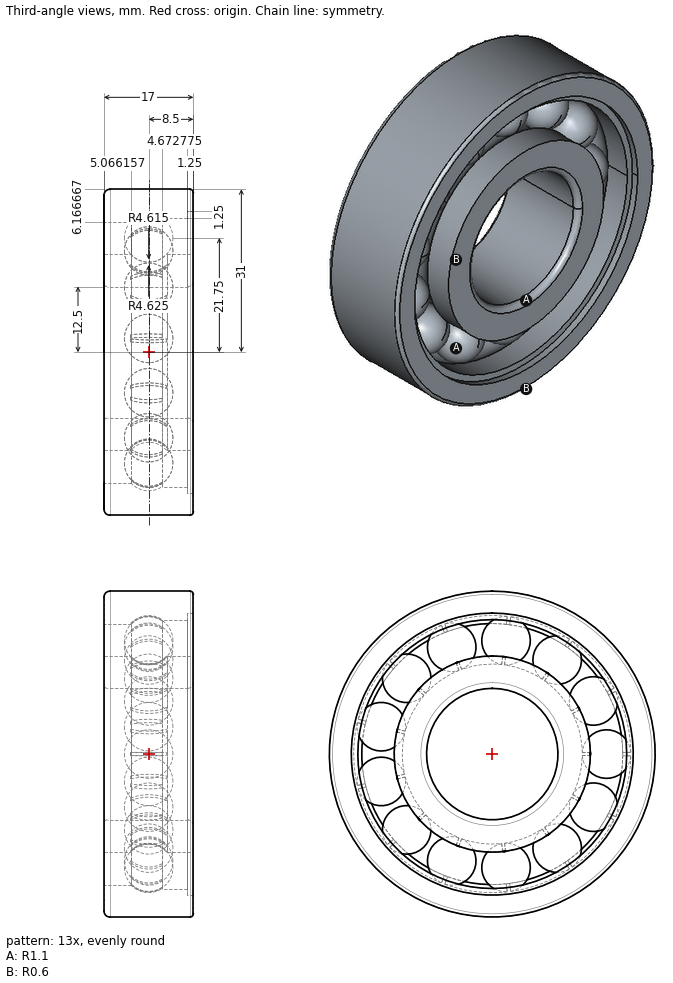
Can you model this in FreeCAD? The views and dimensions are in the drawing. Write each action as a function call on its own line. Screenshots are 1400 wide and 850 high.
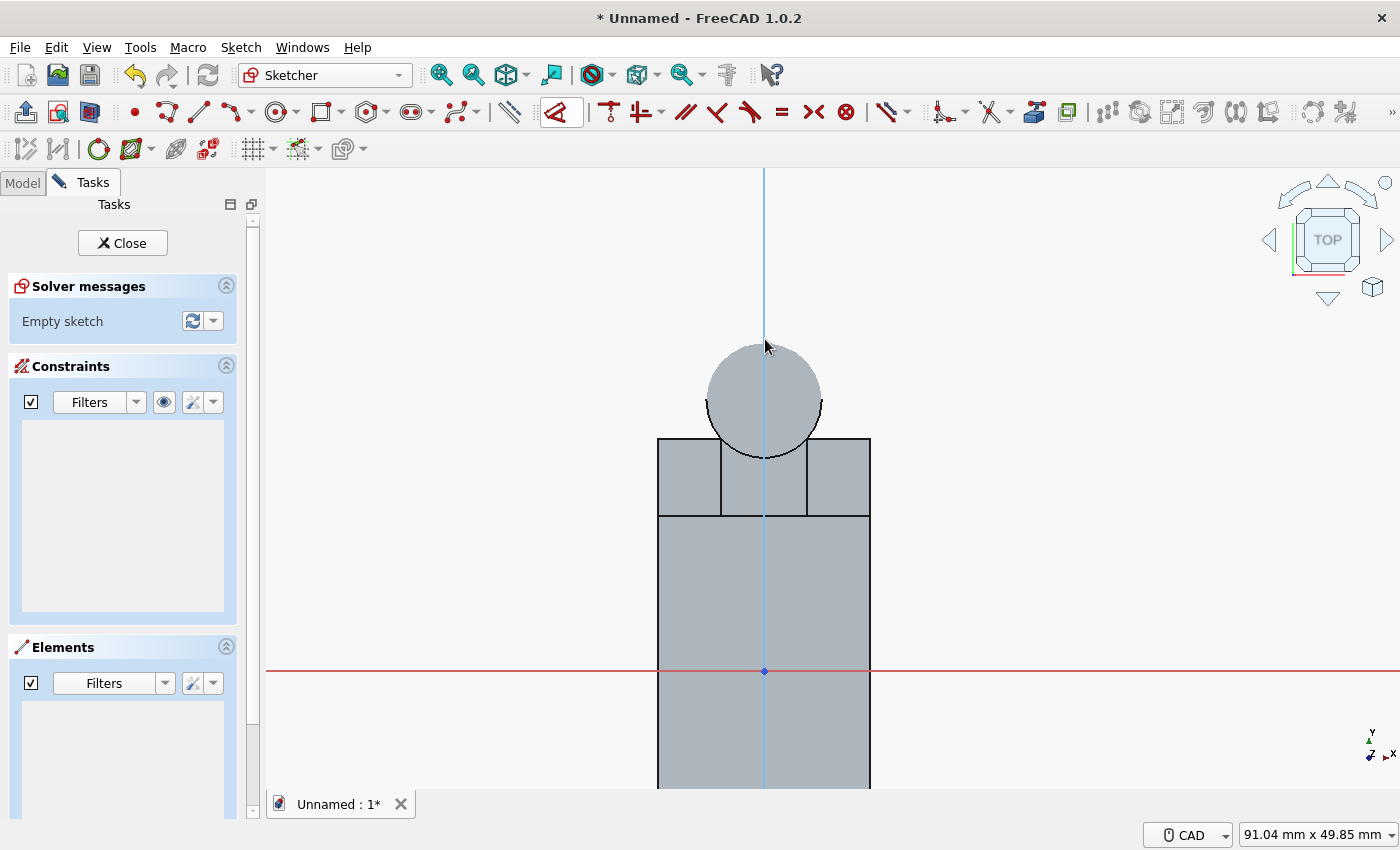
click(168, 112)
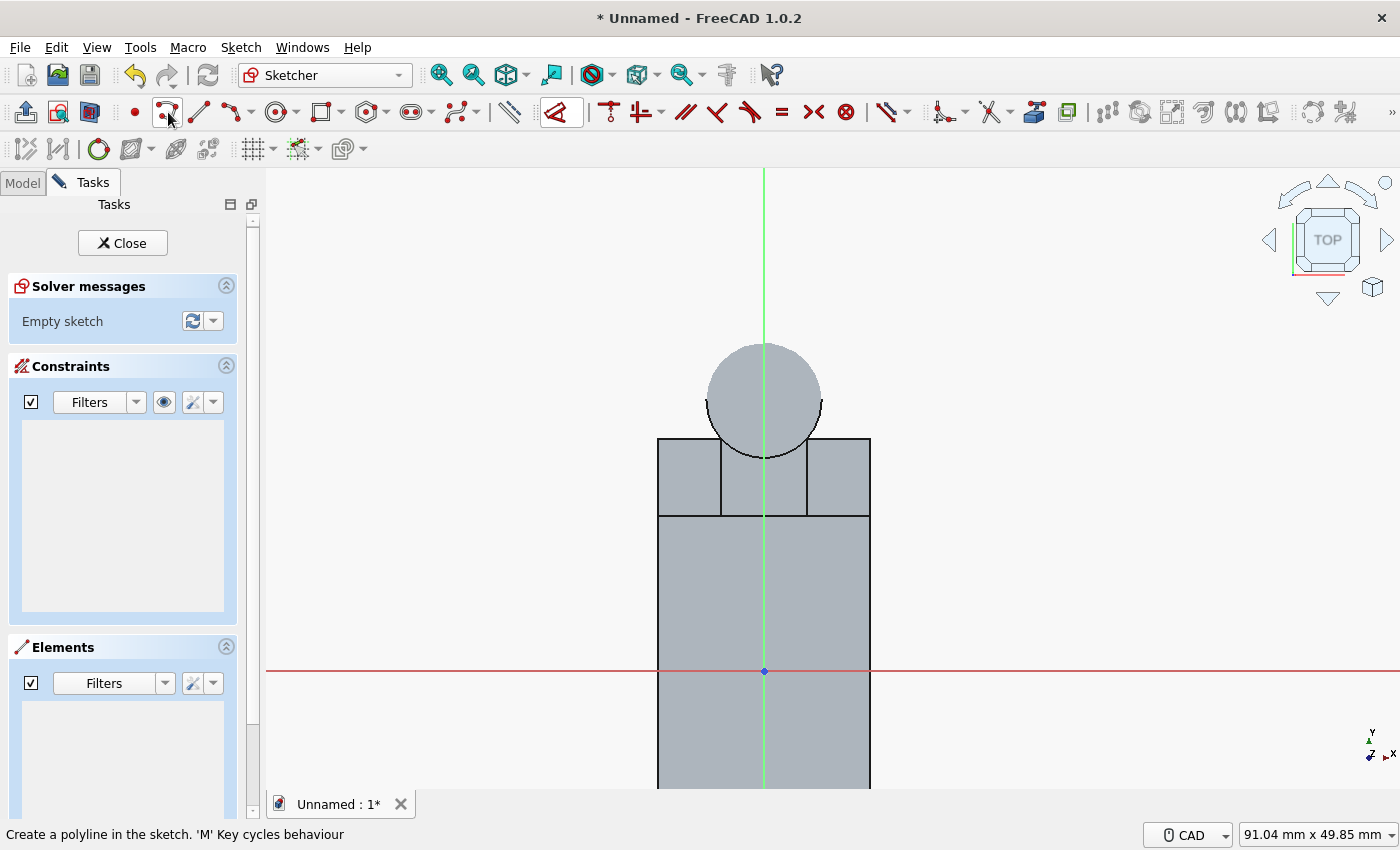
click(796, 353)
click(854, 353)
click(854, 337)
click(870, 337)
click(870, 285)
click(658, 285)
click(658, 362)
click(721, 362)
right_click(721, 362)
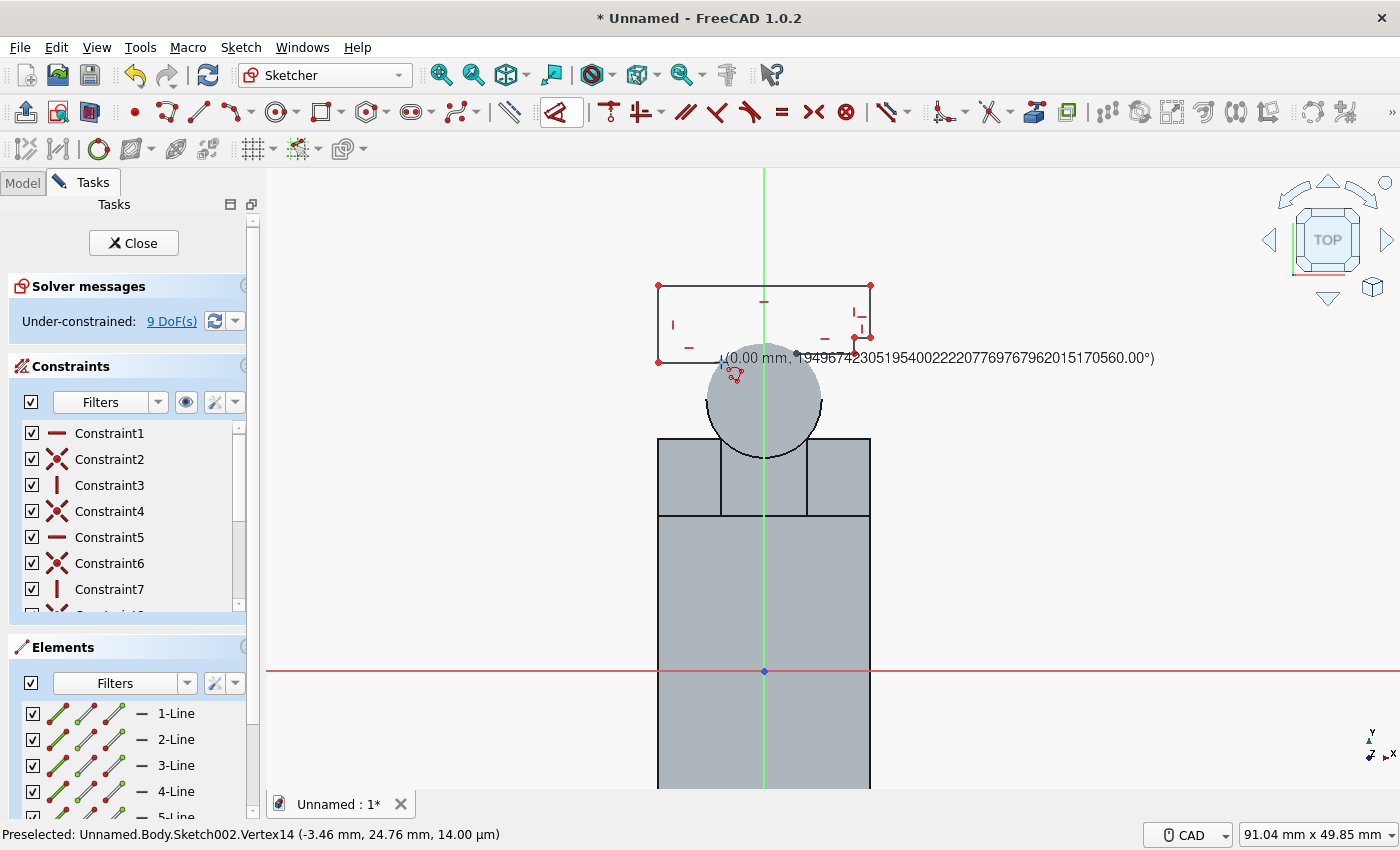
key(g)
key(3)
key(a)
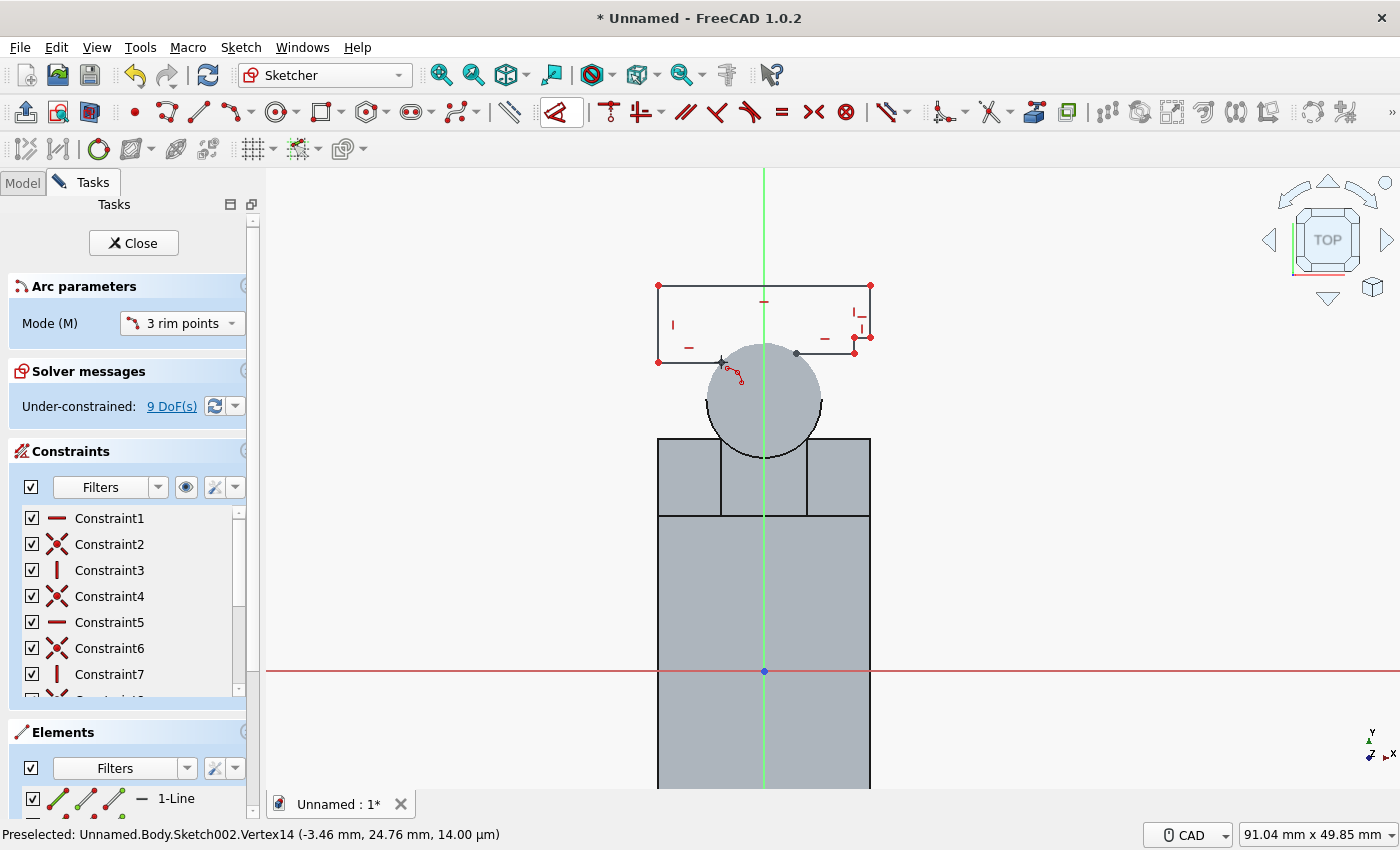
click(721, 363)
click(796, 354)
click(749, 345)
key(Escape)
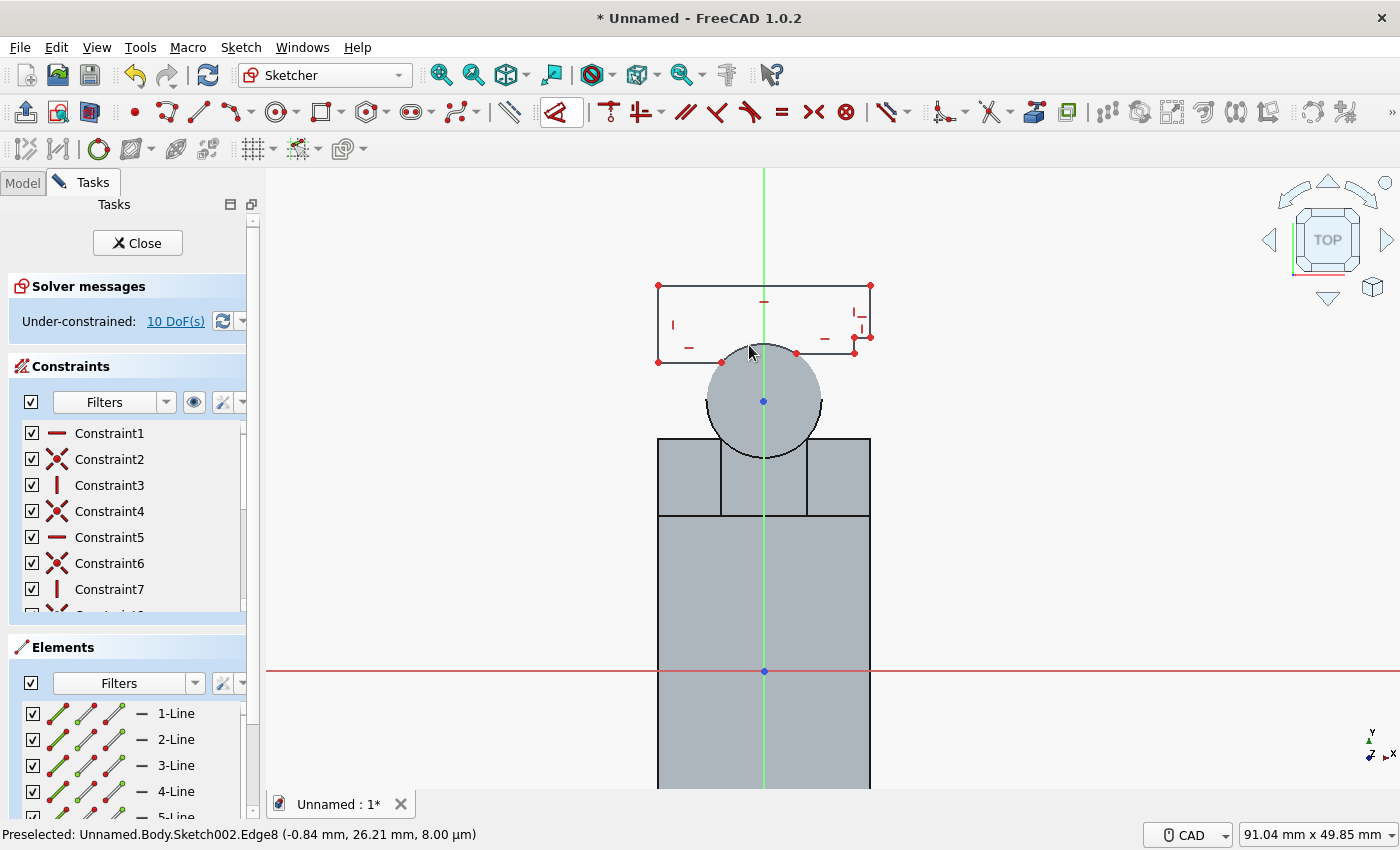
click(764, 402)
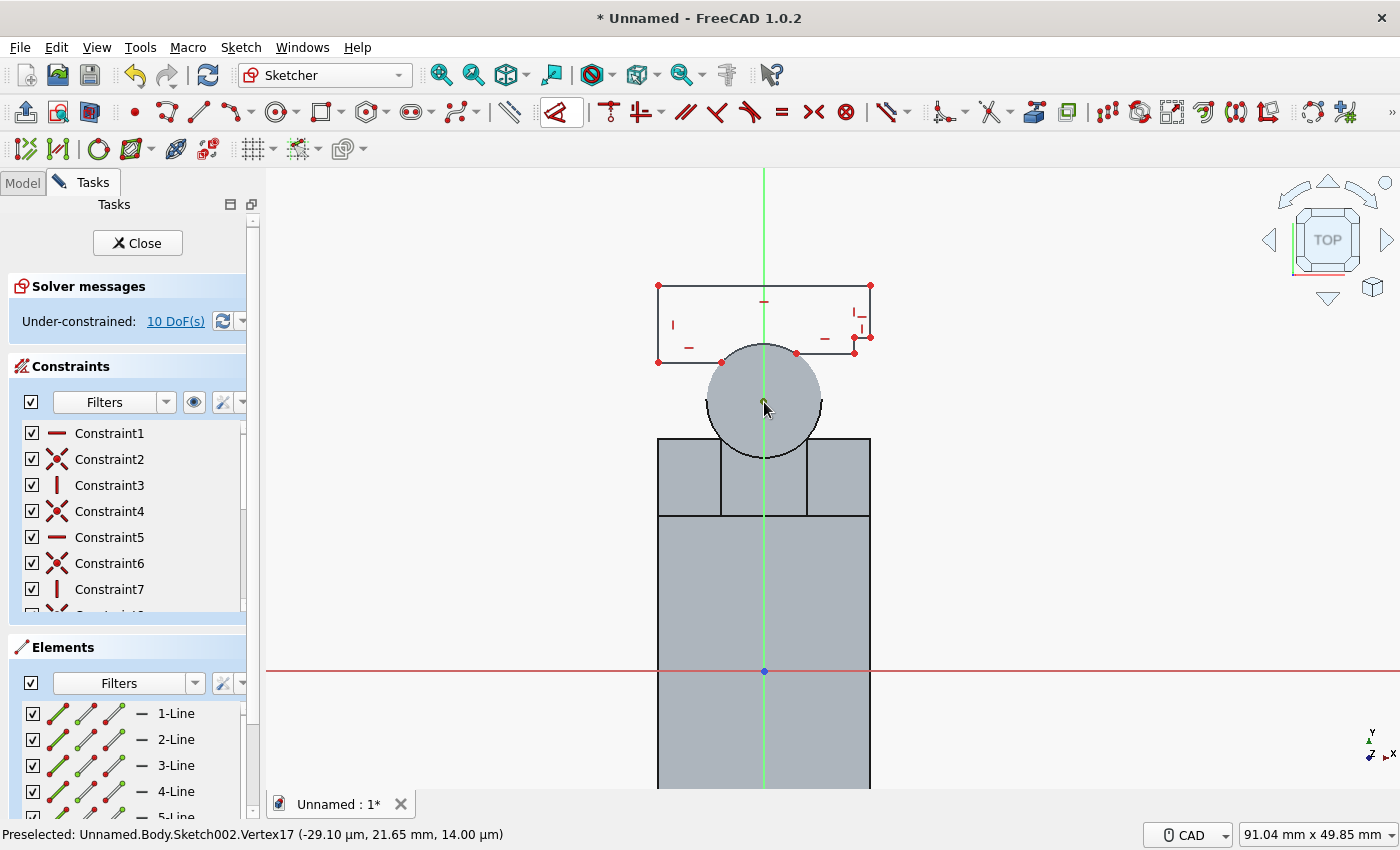
click(764, 721)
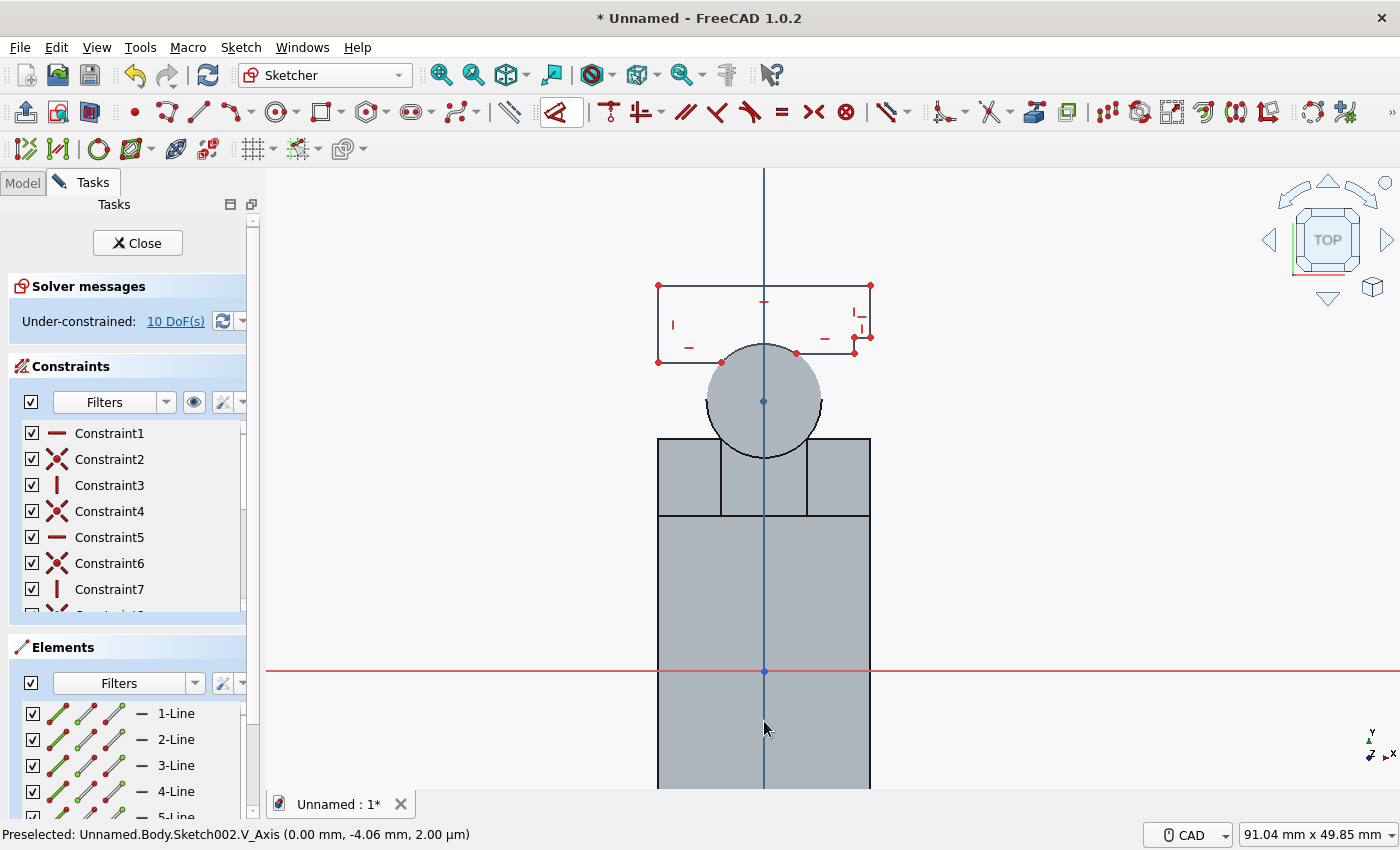
key(c)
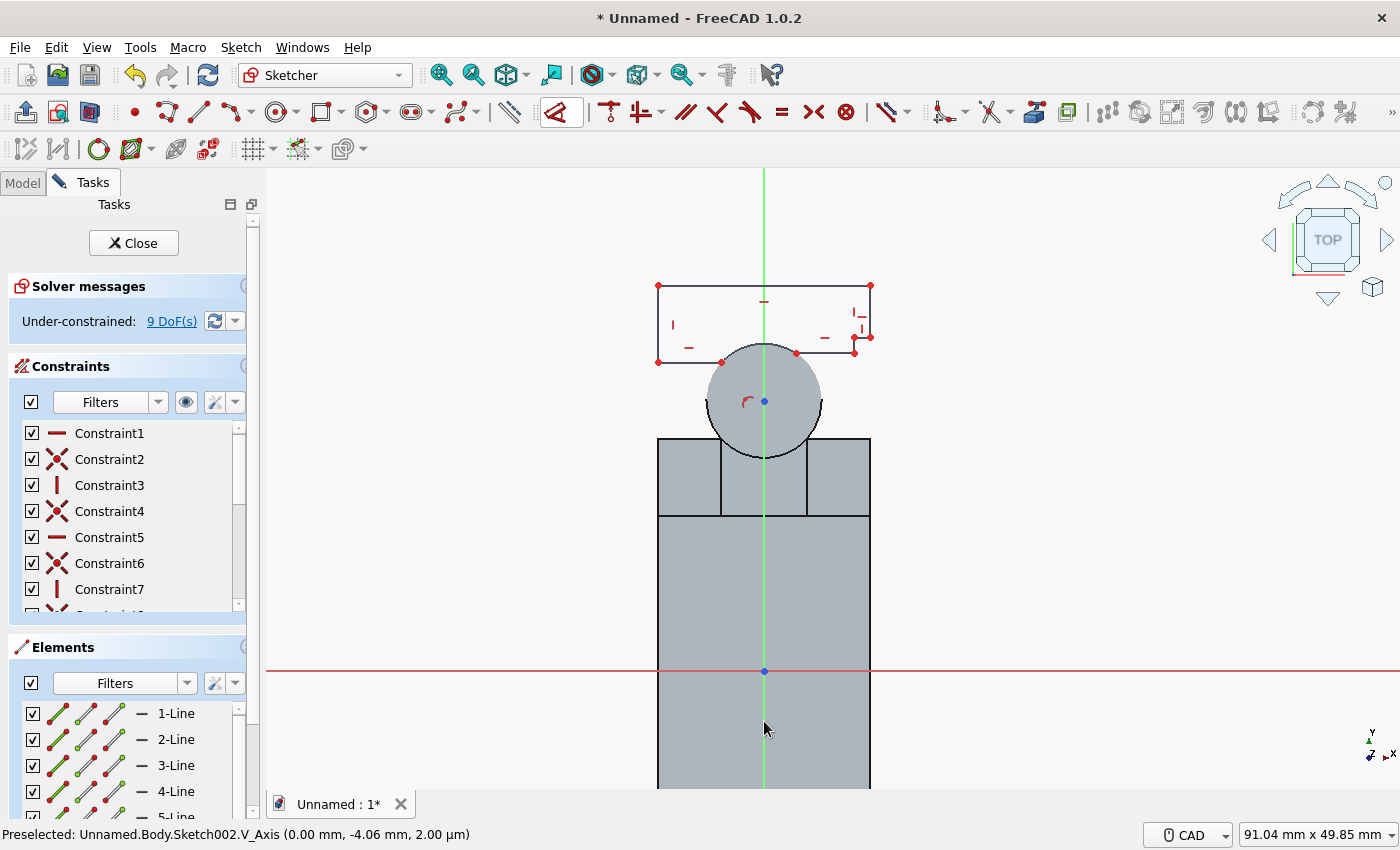
scroll(773, 345, up, 3)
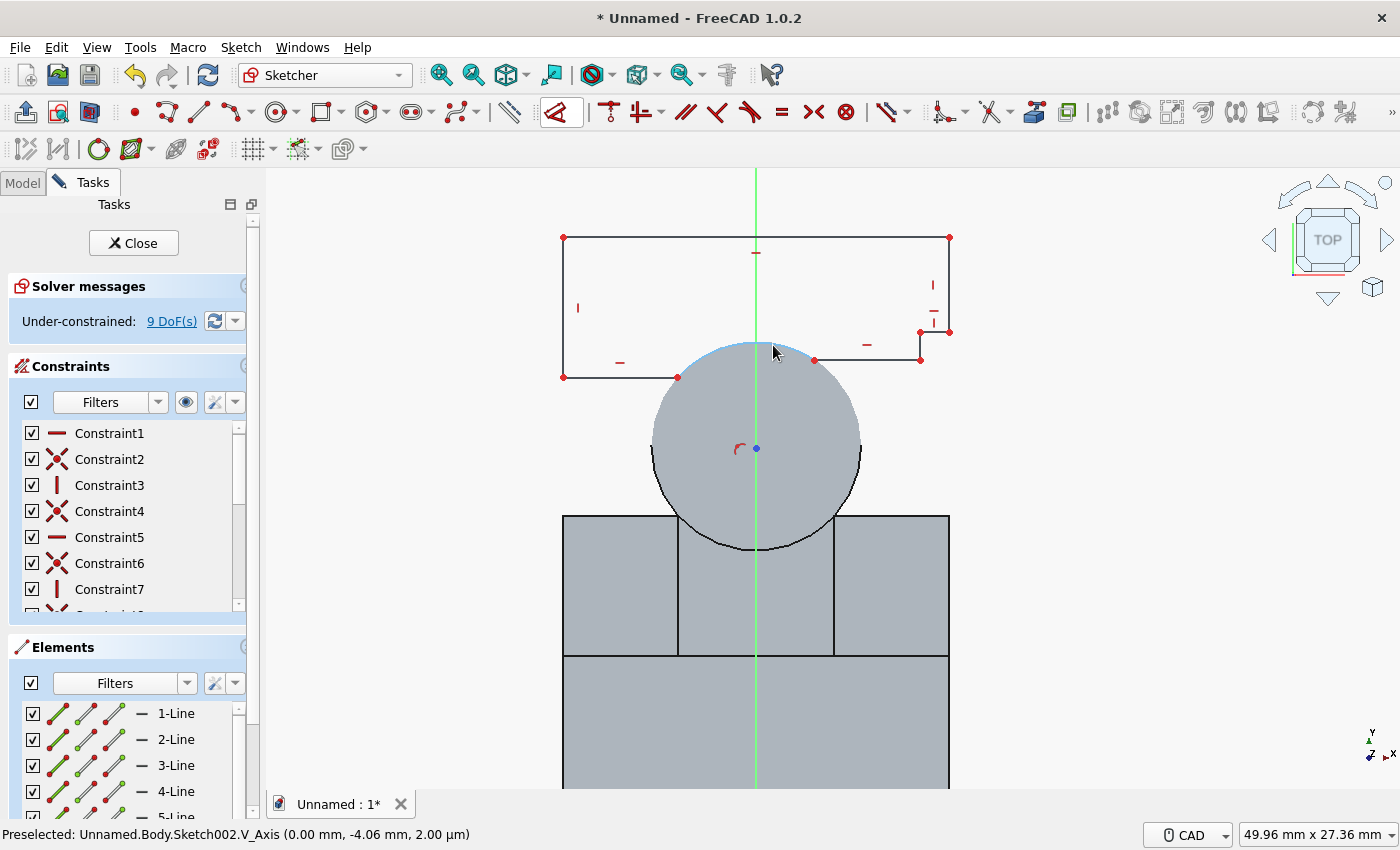
click(773, 344)